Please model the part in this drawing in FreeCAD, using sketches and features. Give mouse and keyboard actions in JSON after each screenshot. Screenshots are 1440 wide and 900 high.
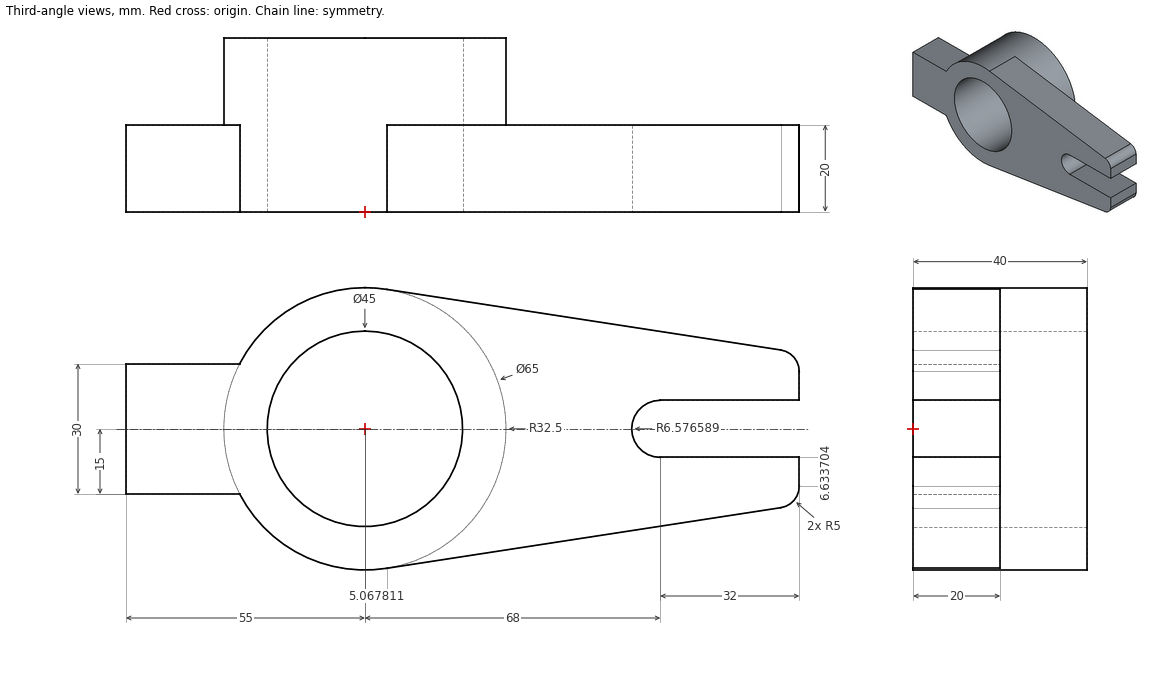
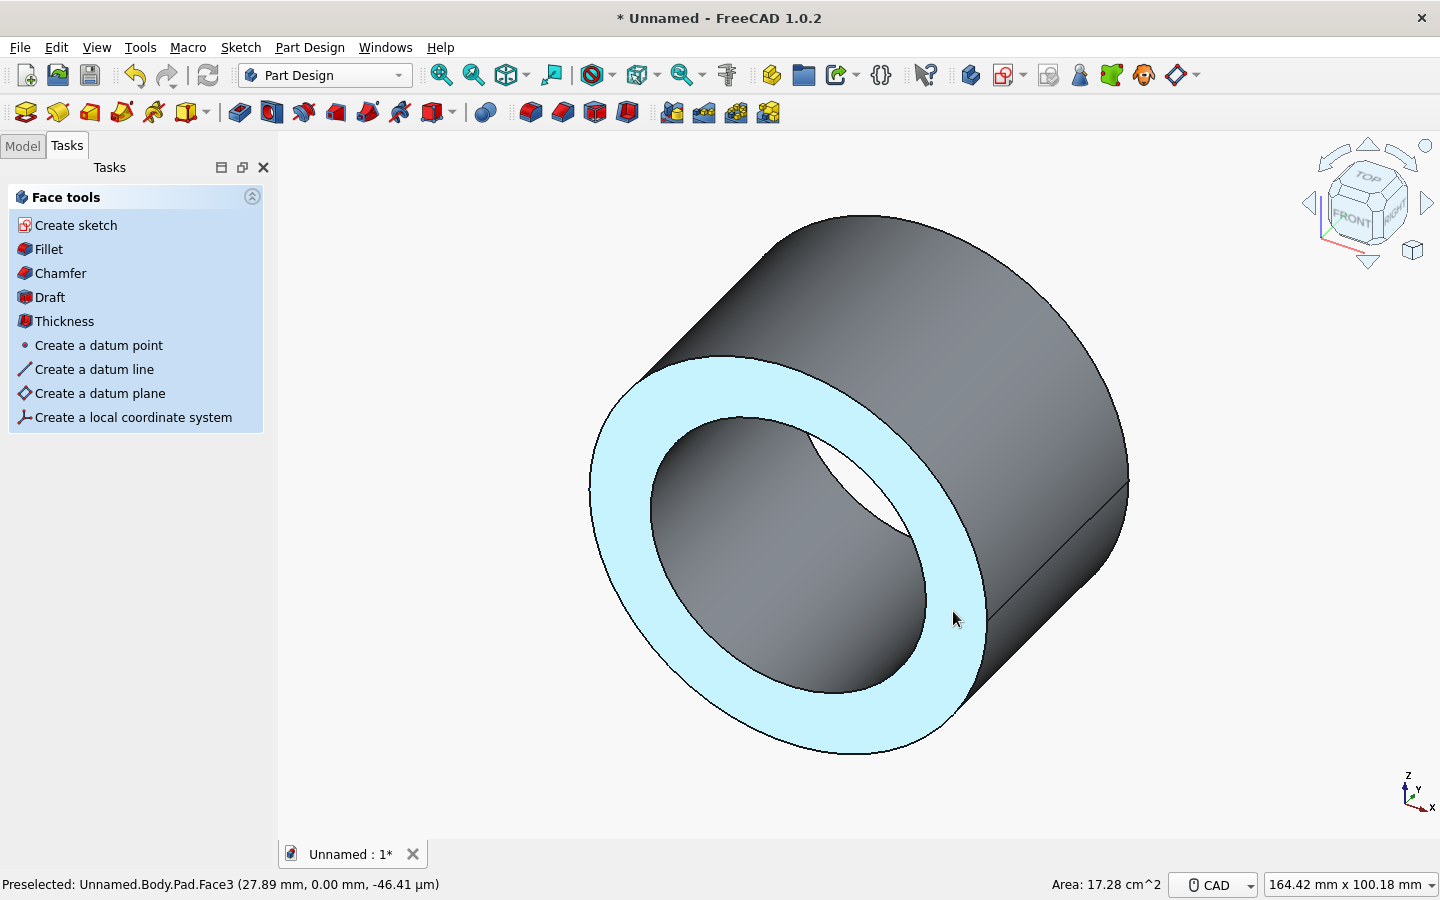
{"action": "left_click", "coordinate": [1004, 76]}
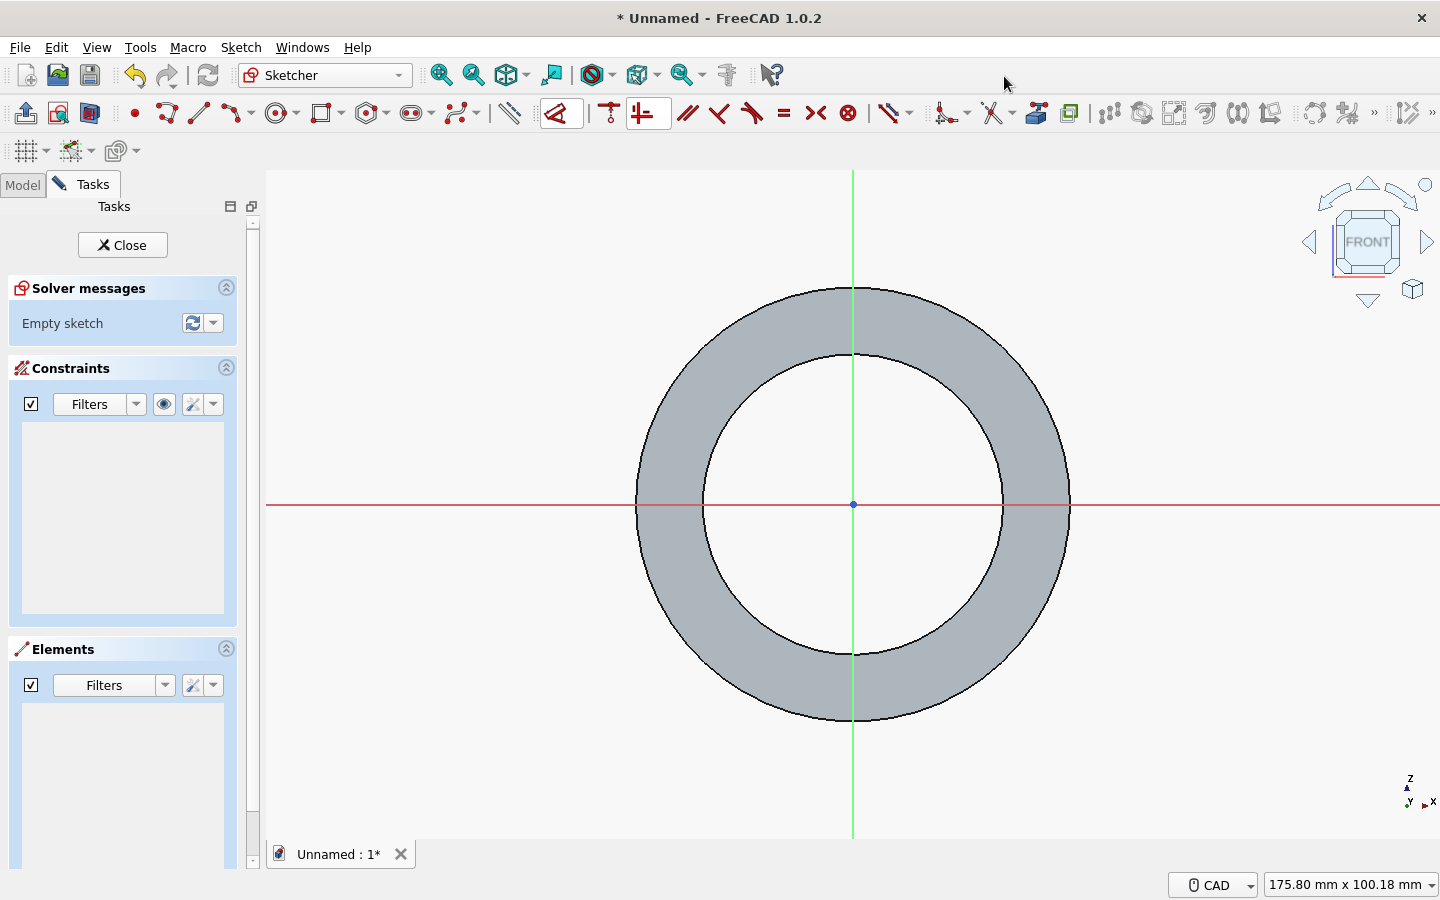
{"action": "scroll", "coordinate": [294, 504], "scroll_direction": "down", "scroll_amount": 2}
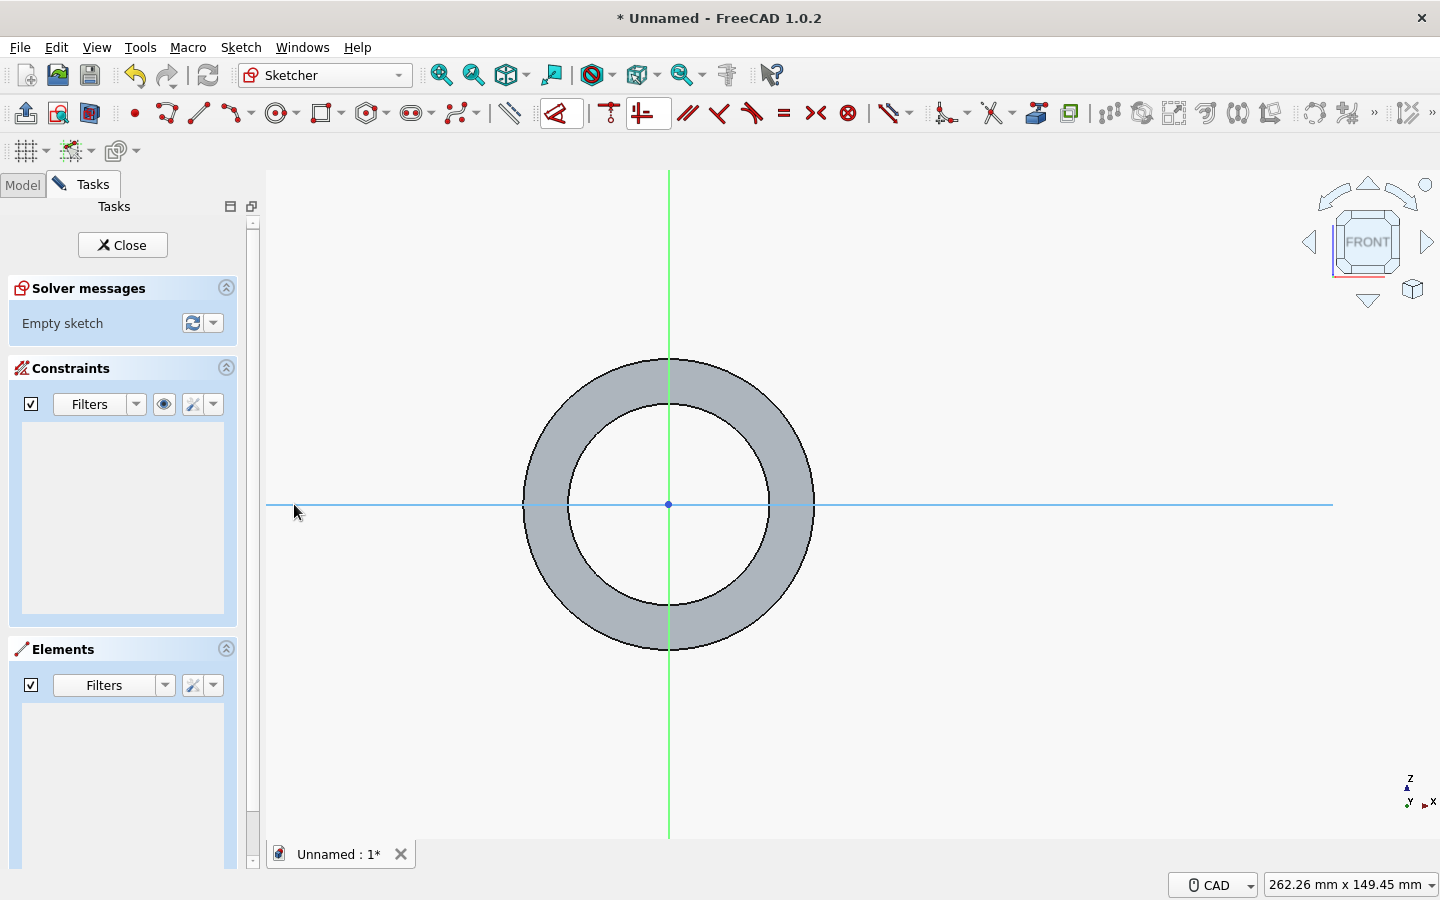
{"action": "scroll", "coordinate": [1112, 505], "scroll_direction": "up", "scroll_amount": 2}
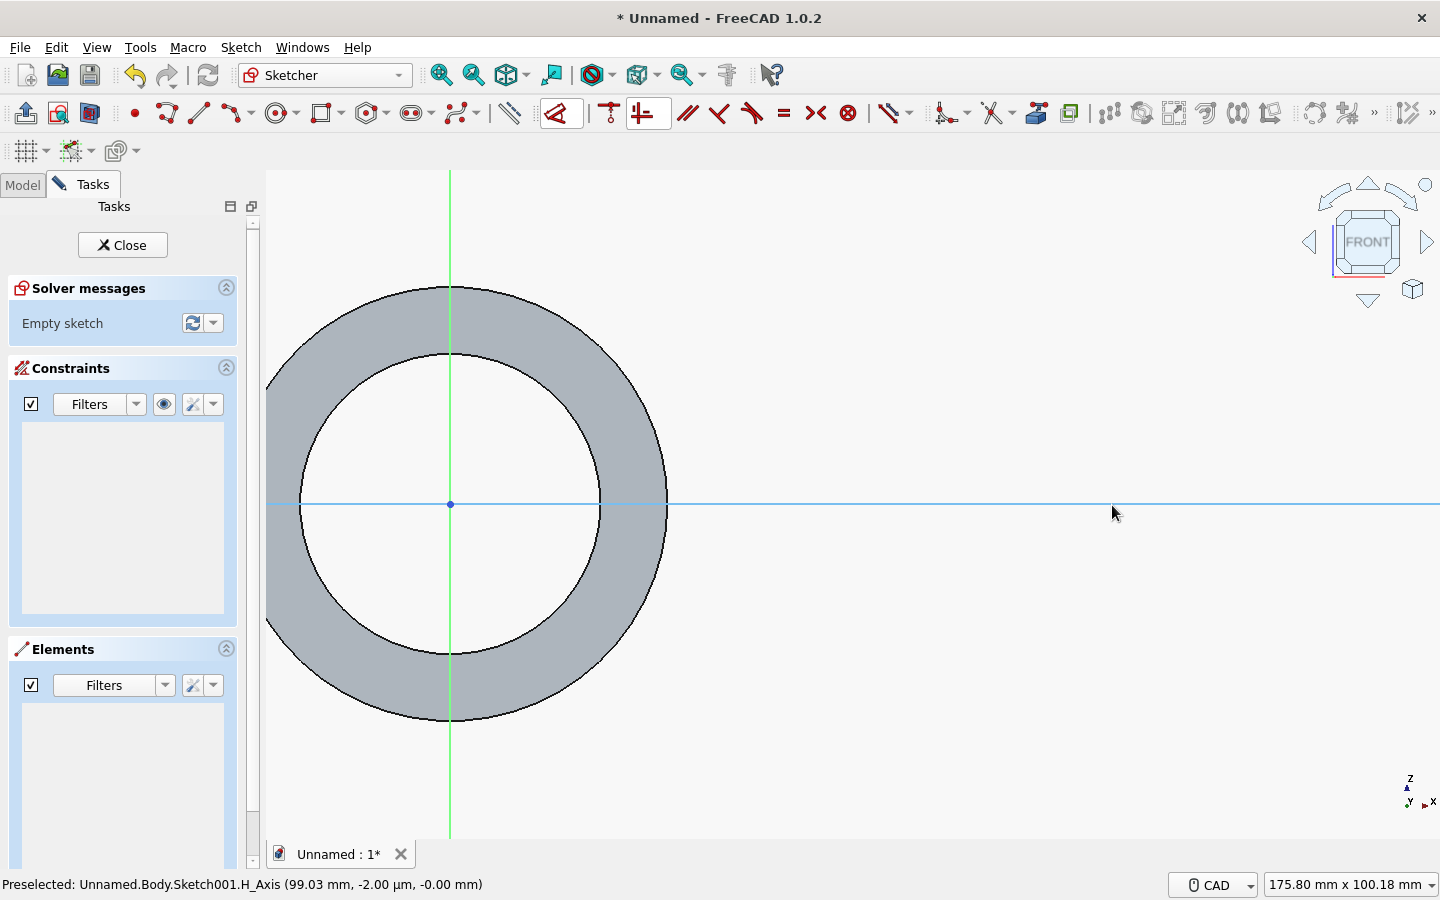
{"action": "left_click", "coordinate": [168, 114]}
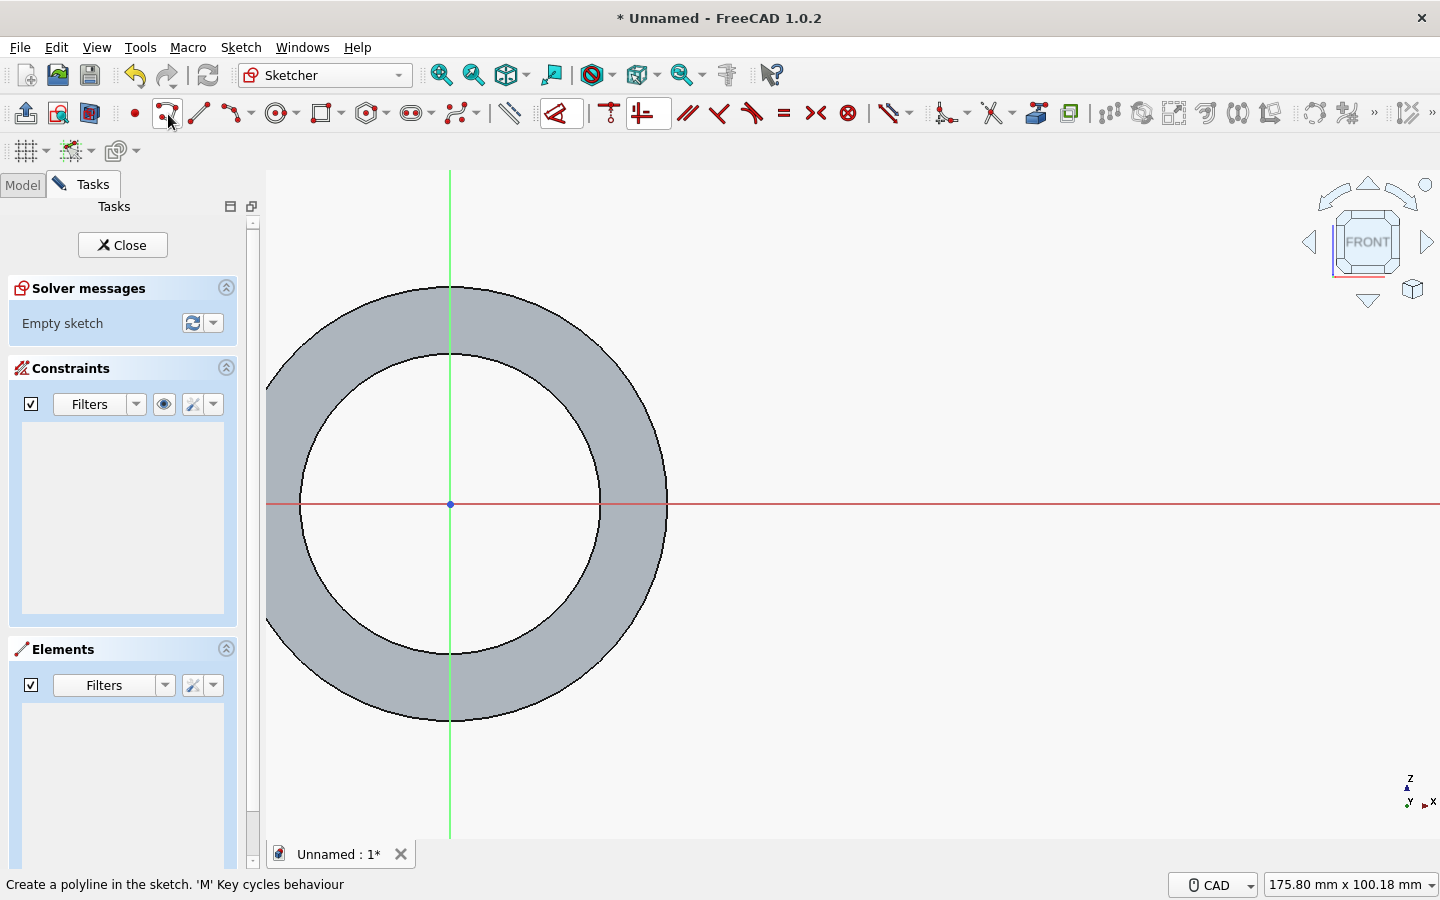
{"action": "left_click", "coordinate": [904, 548]}
{"action": "left_click", "coordinate": [1118, 548]}
{"action": "left_click", "coordinate": [1118, 592]}
{"action": "right_click", "coordinate": [1118, 592]}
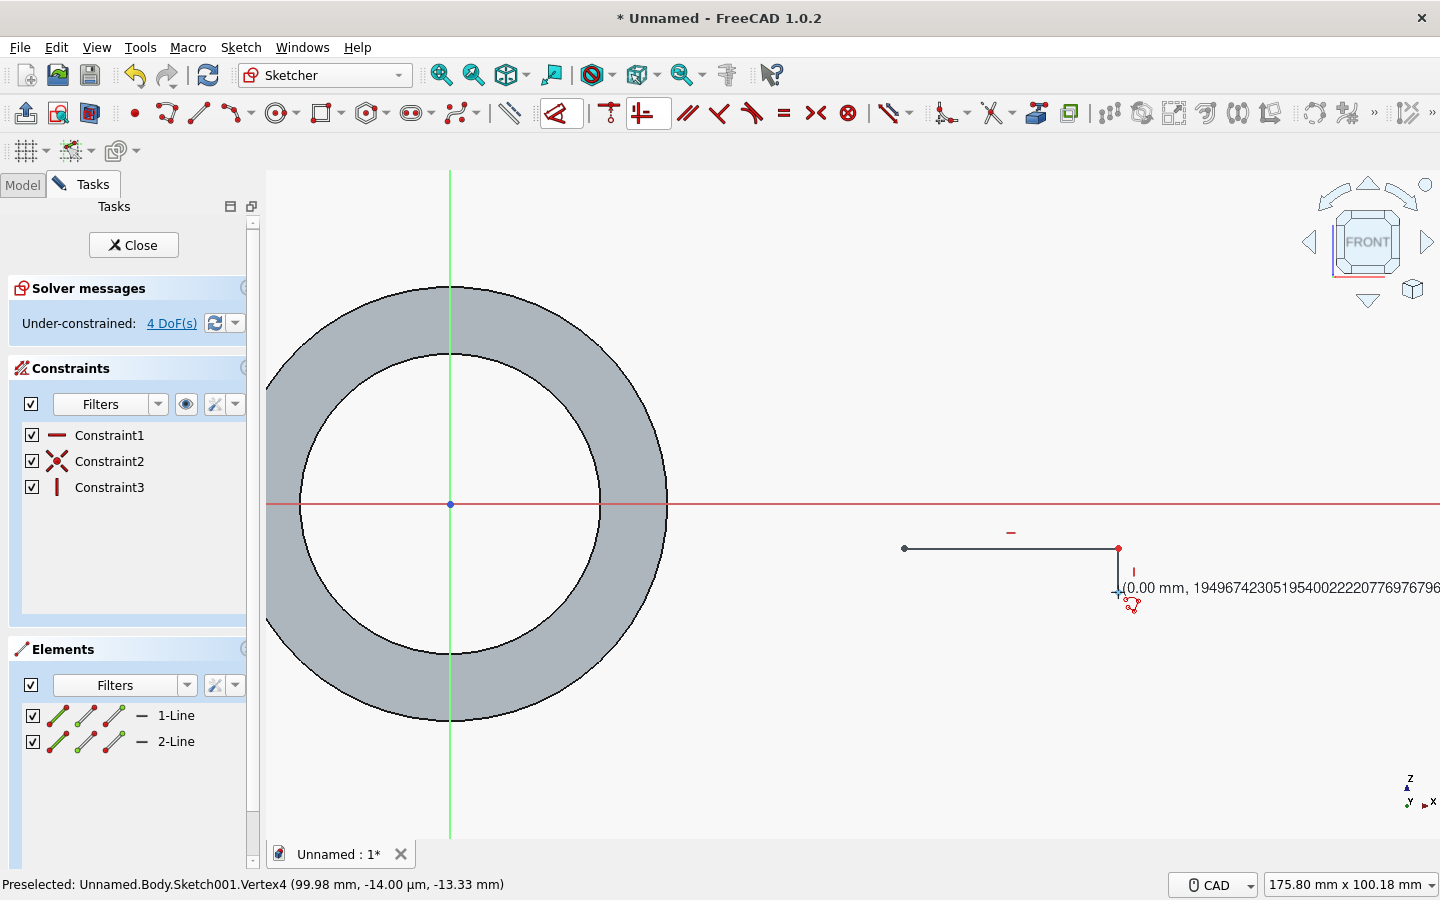
{"action": "left_click", "coordinate": [200, 114]}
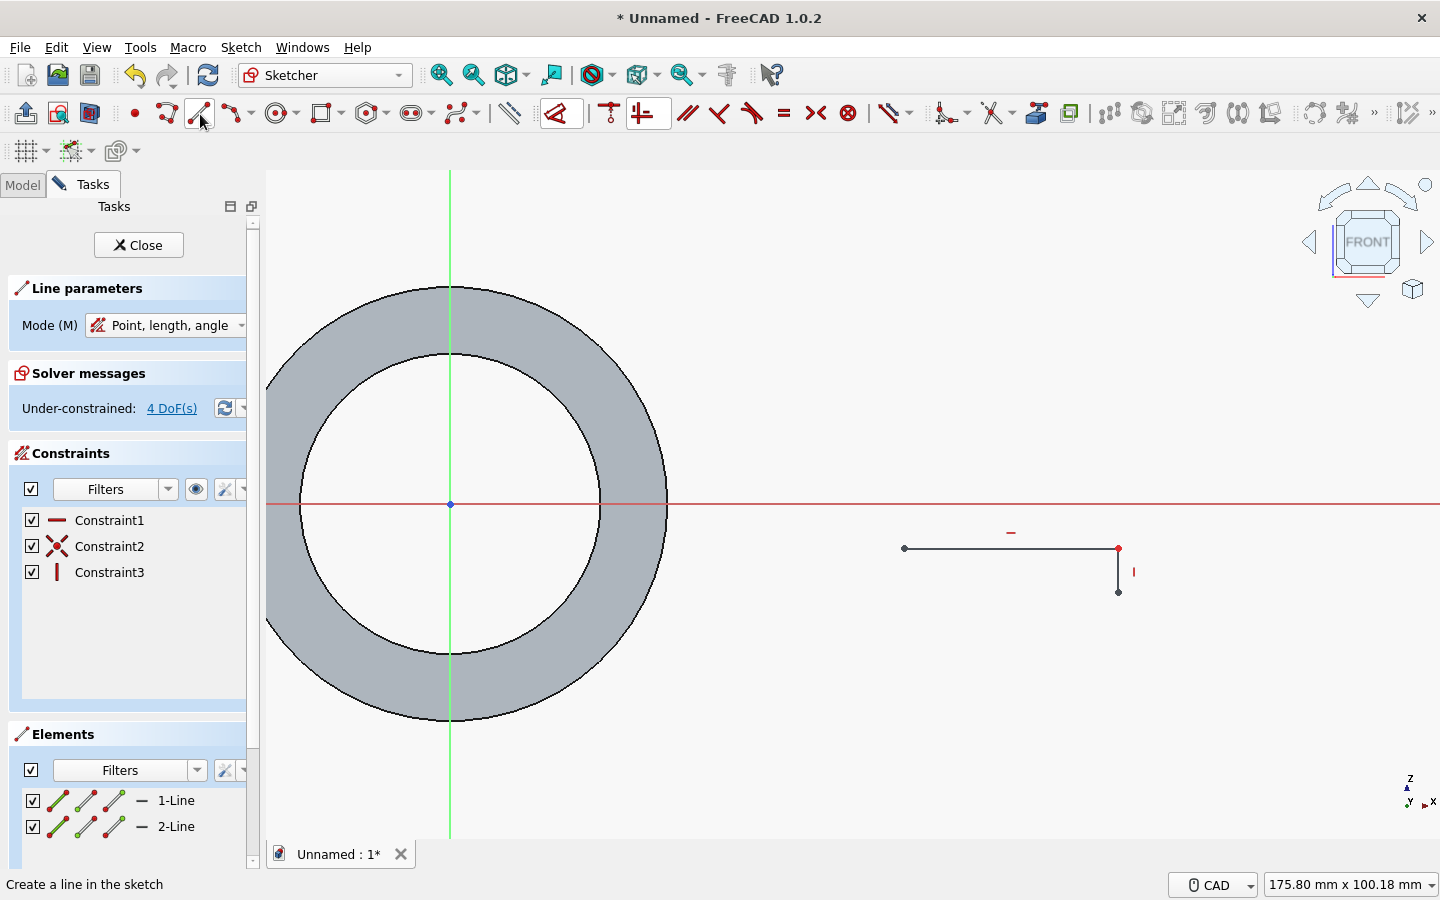
{"action": "left_click", "coordinate": [1090, 625]}
{"action": "left_click", "coordinate": [484, 718]}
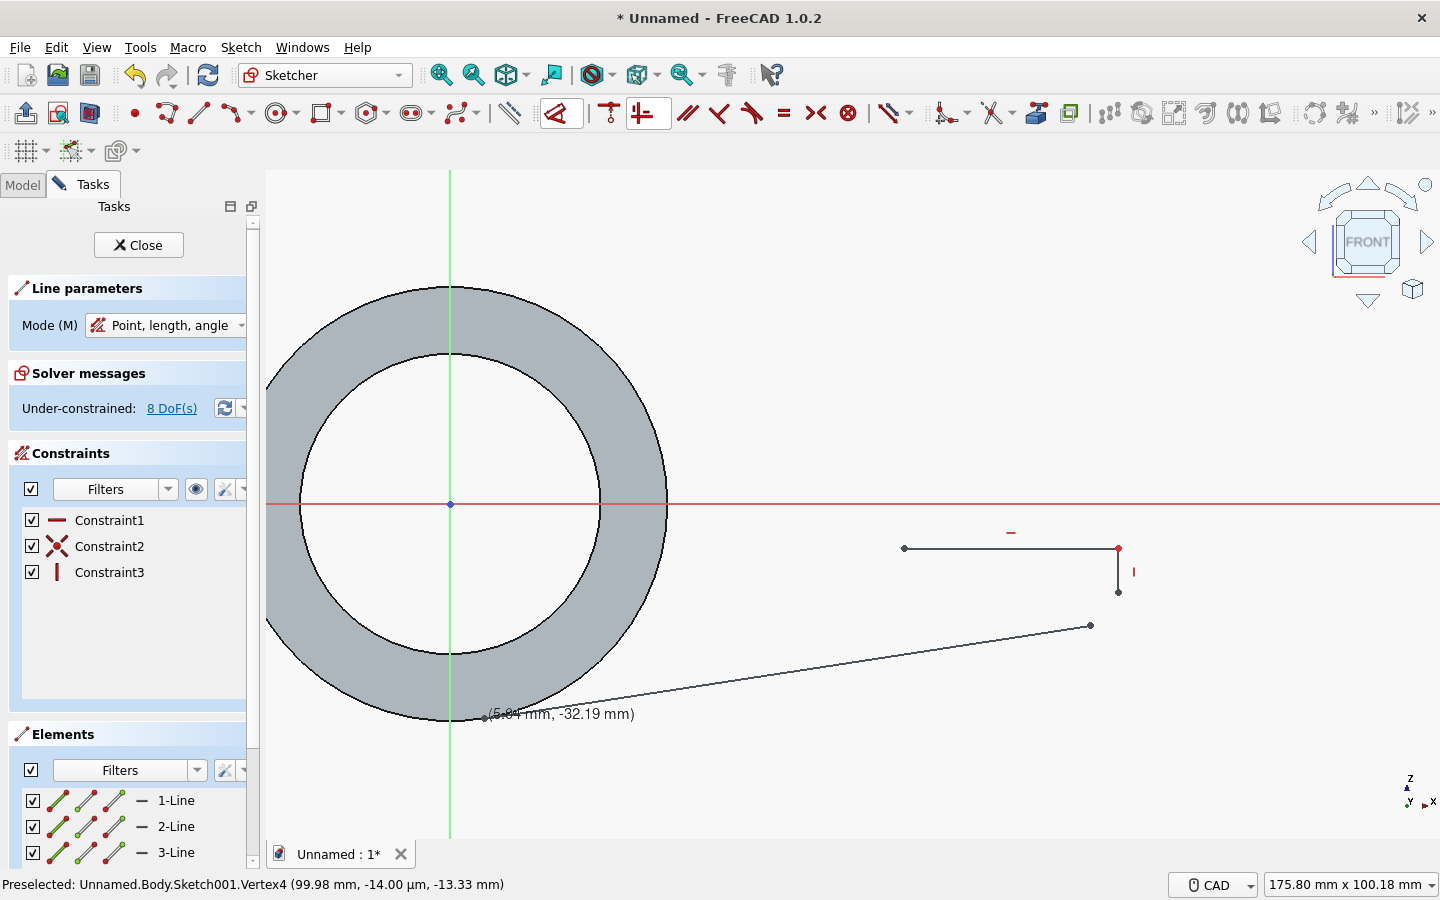
{"action": "left_click", "coordinate": [484, 290]}
{"action": "left_click", "coordinate": [1090, 383]}